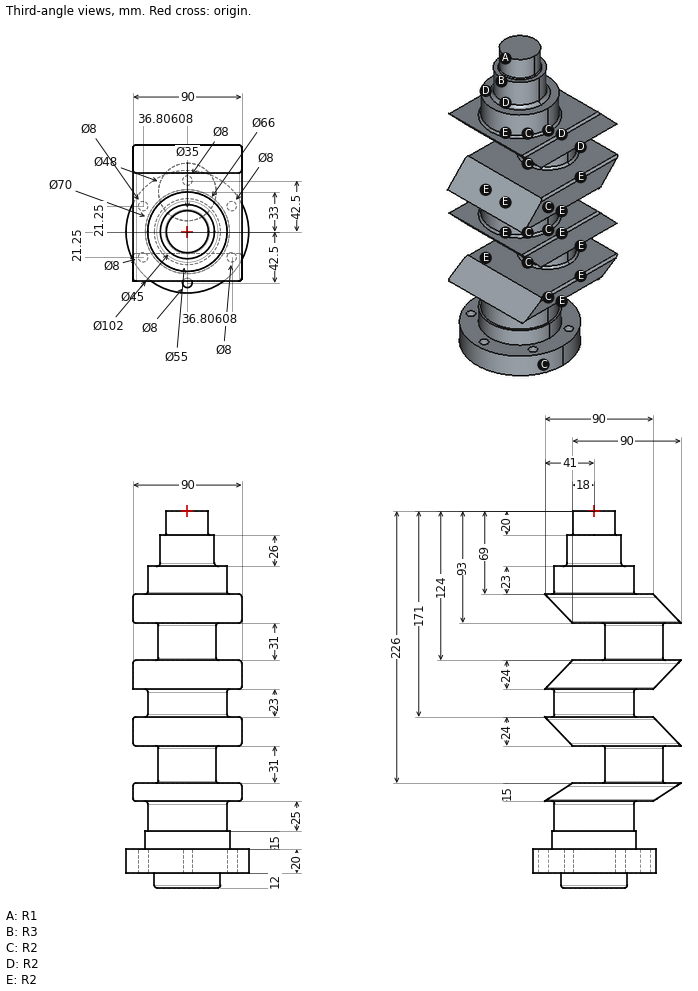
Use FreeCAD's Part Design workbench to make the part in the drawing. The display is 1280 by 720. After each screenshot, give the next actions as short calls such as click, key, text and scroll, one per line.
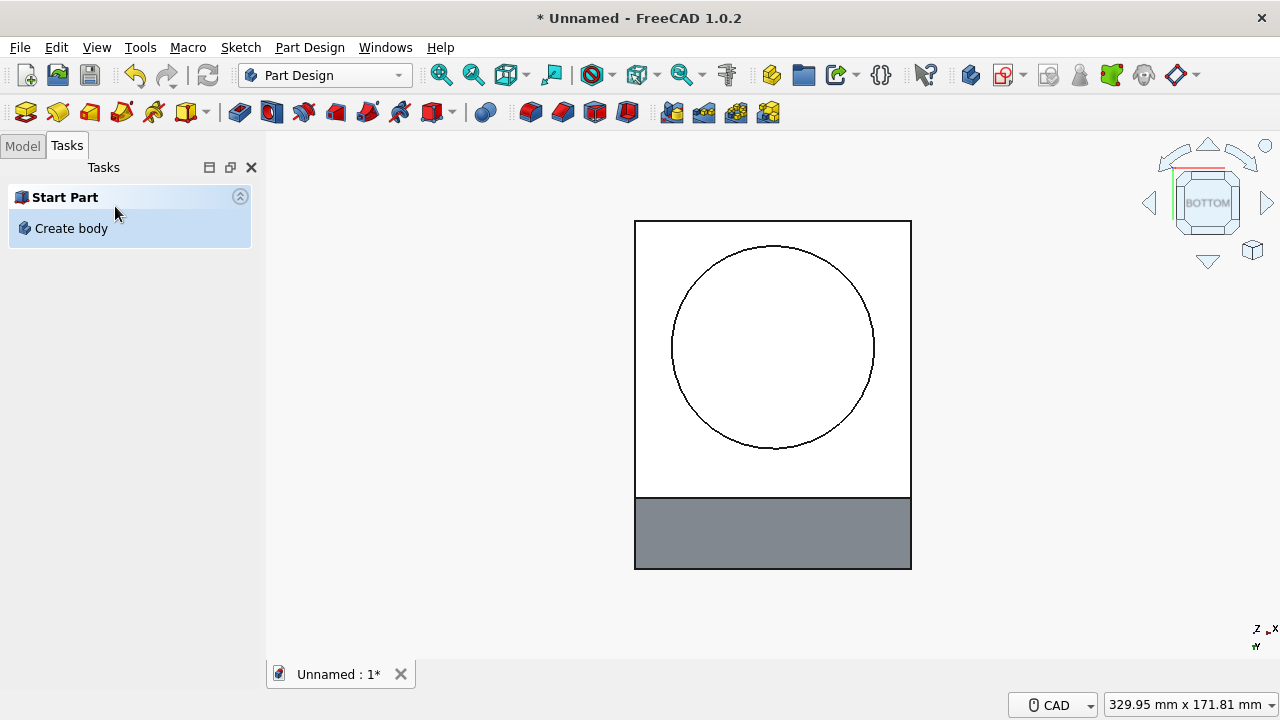
click(1004, 76)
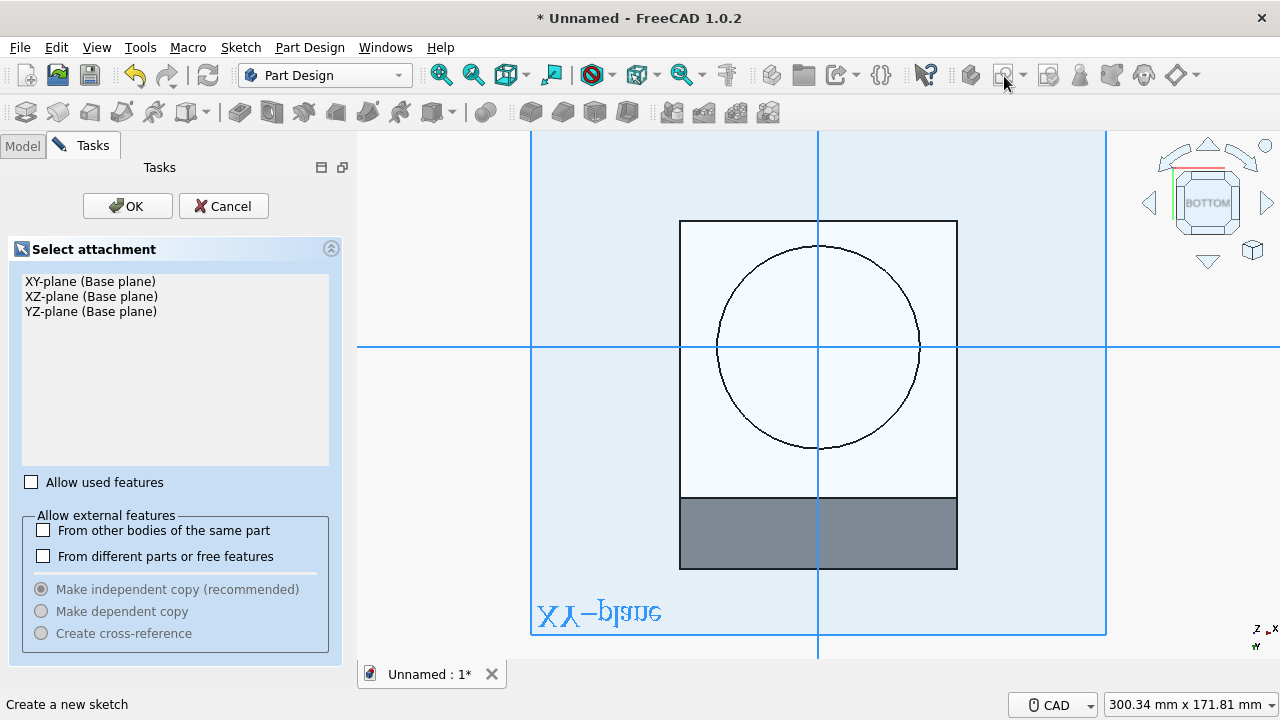
click(82, 312)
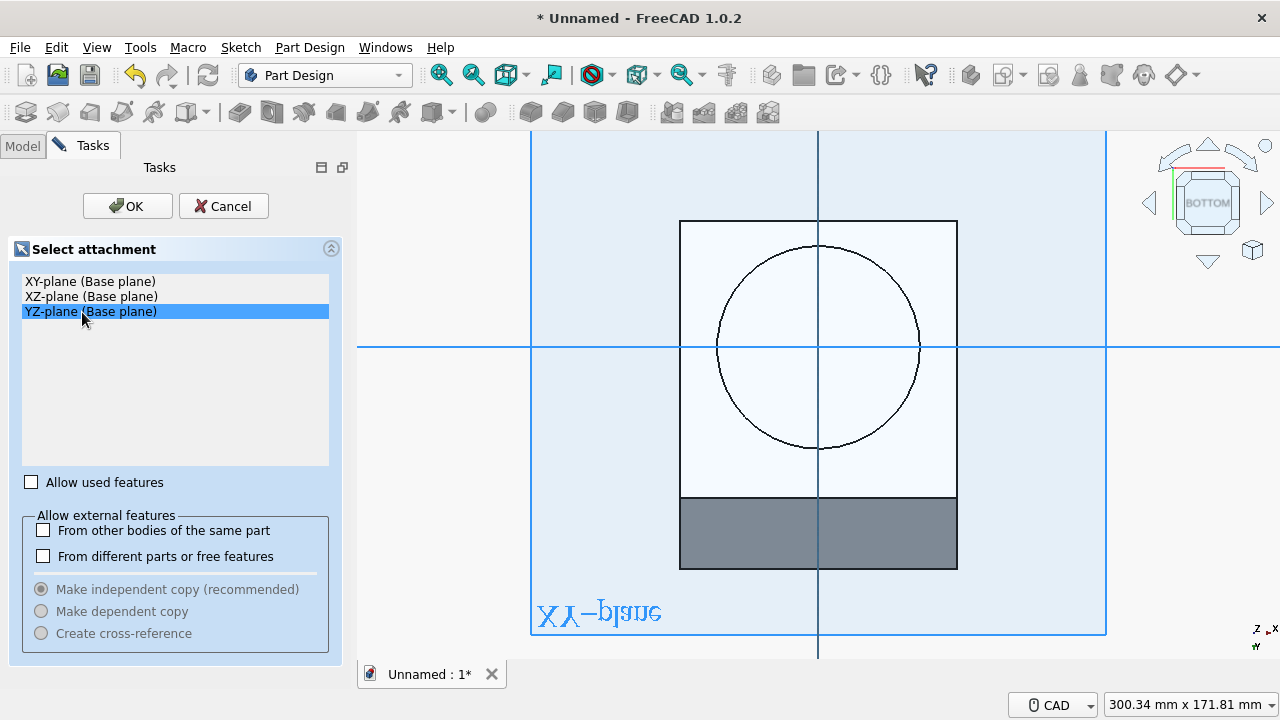
click(128, 206)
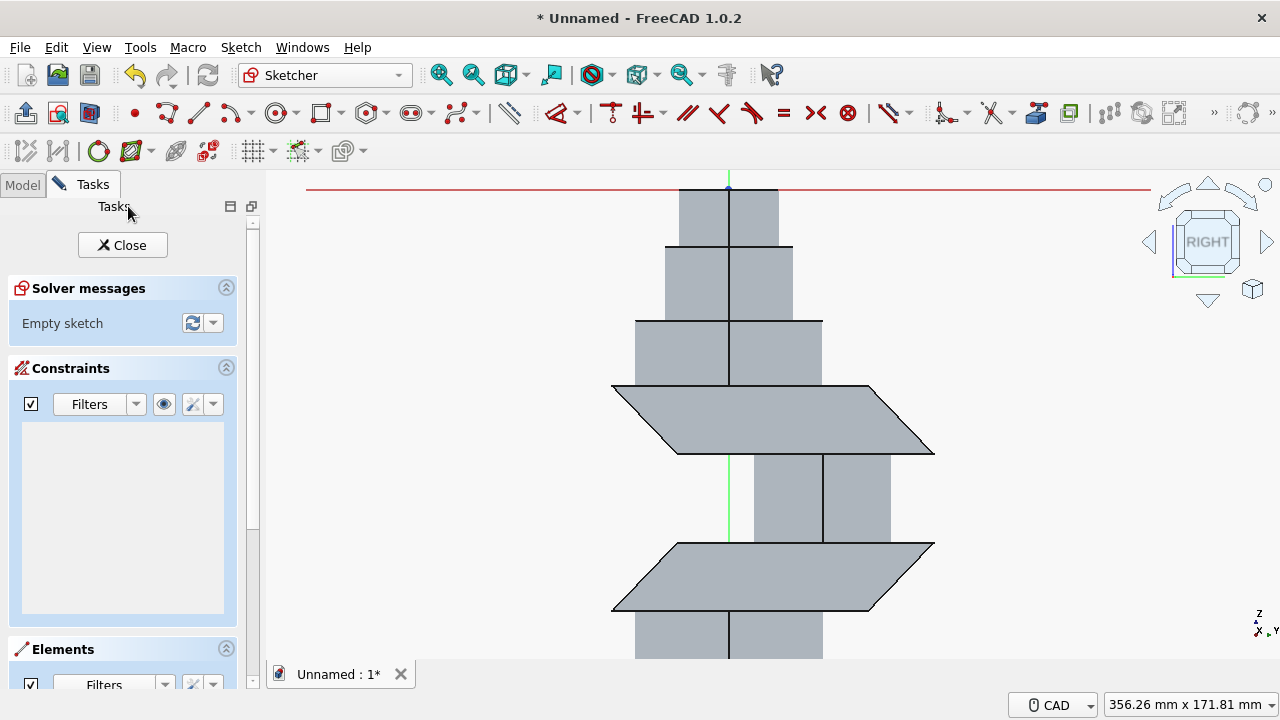
click(90, 114)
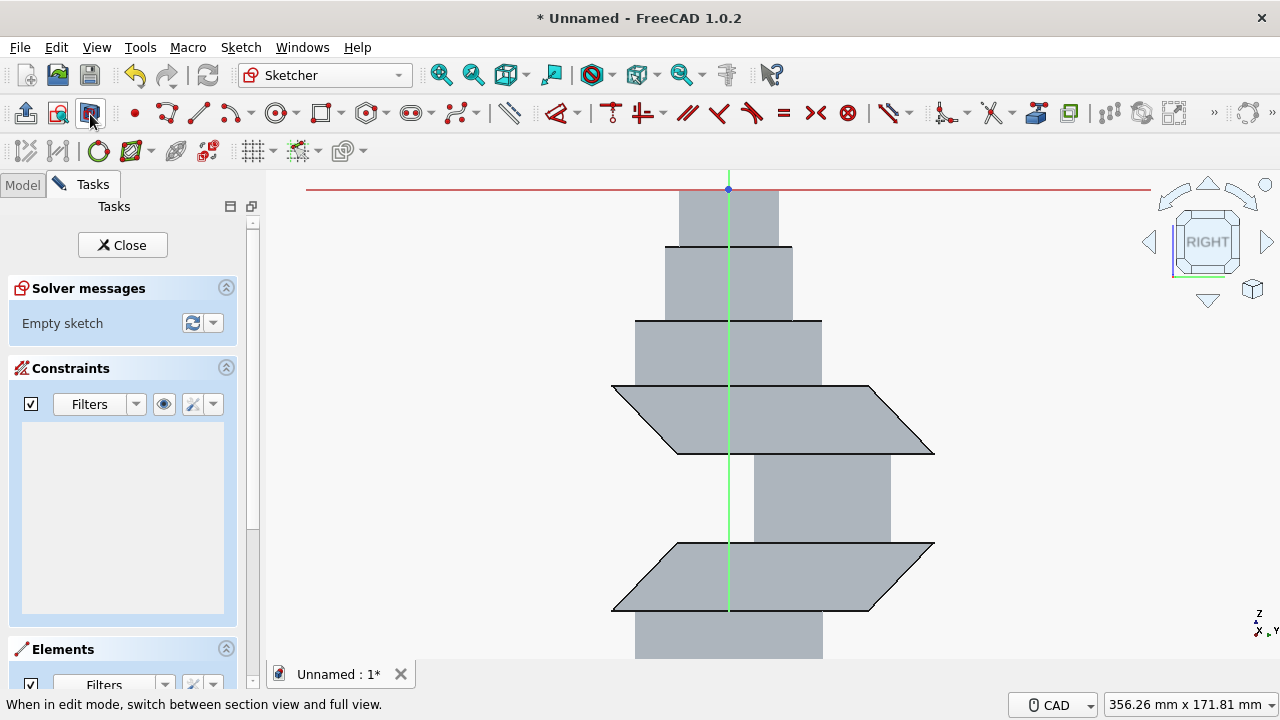
scroll(621, 350, down, 3)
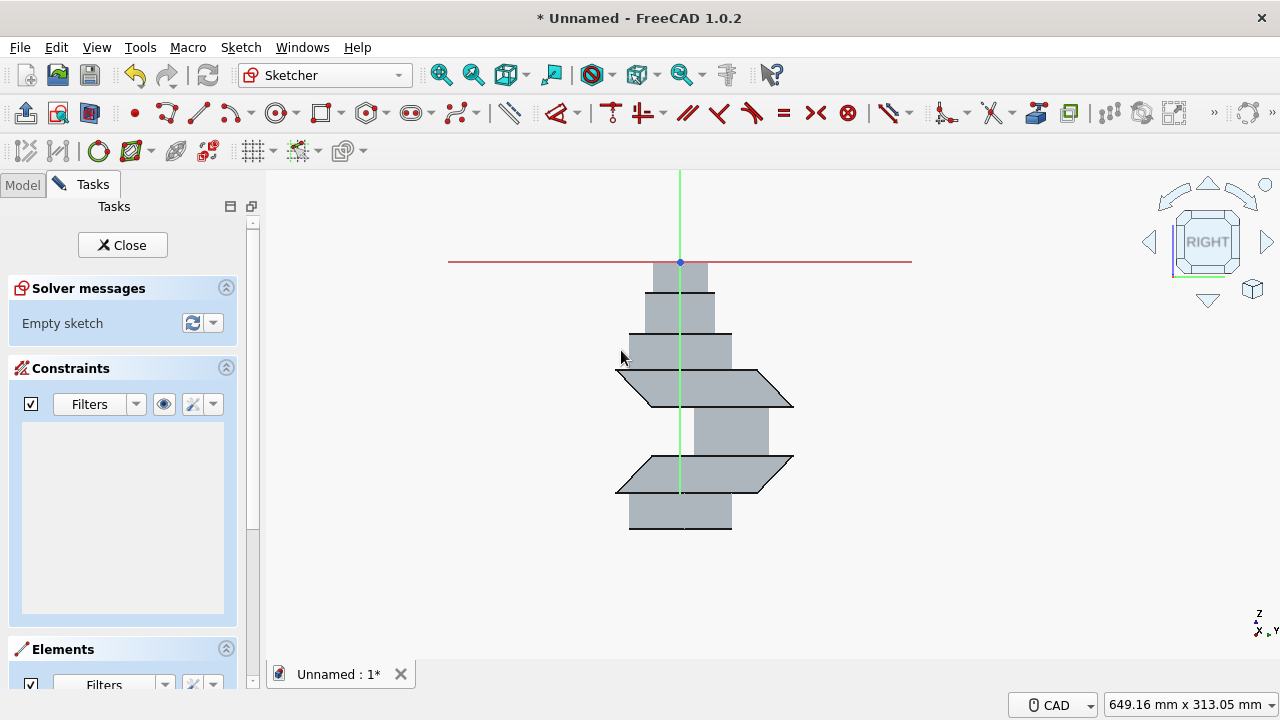
click(168, 114)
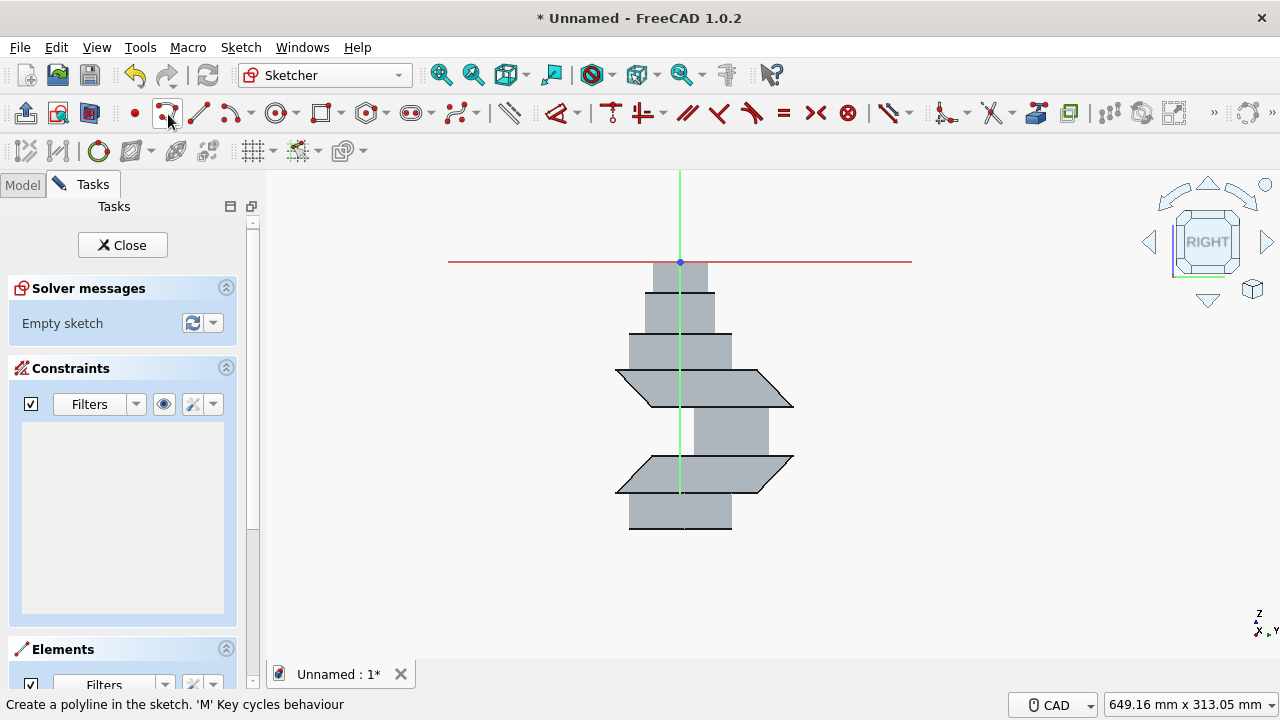
click(616, 529)
click(652, 567)
click(793, 567)
click(757, 529)
click(616, 530)
key(Escape)
key(Escape)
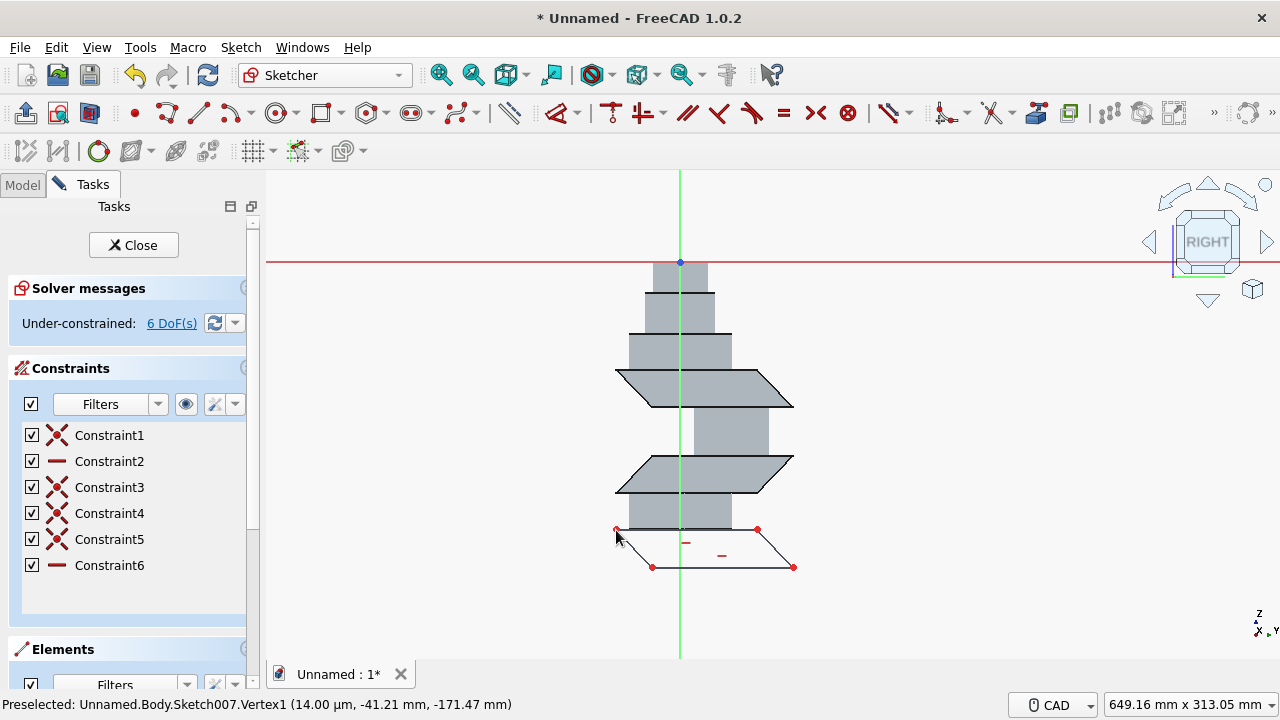
click(556, 114)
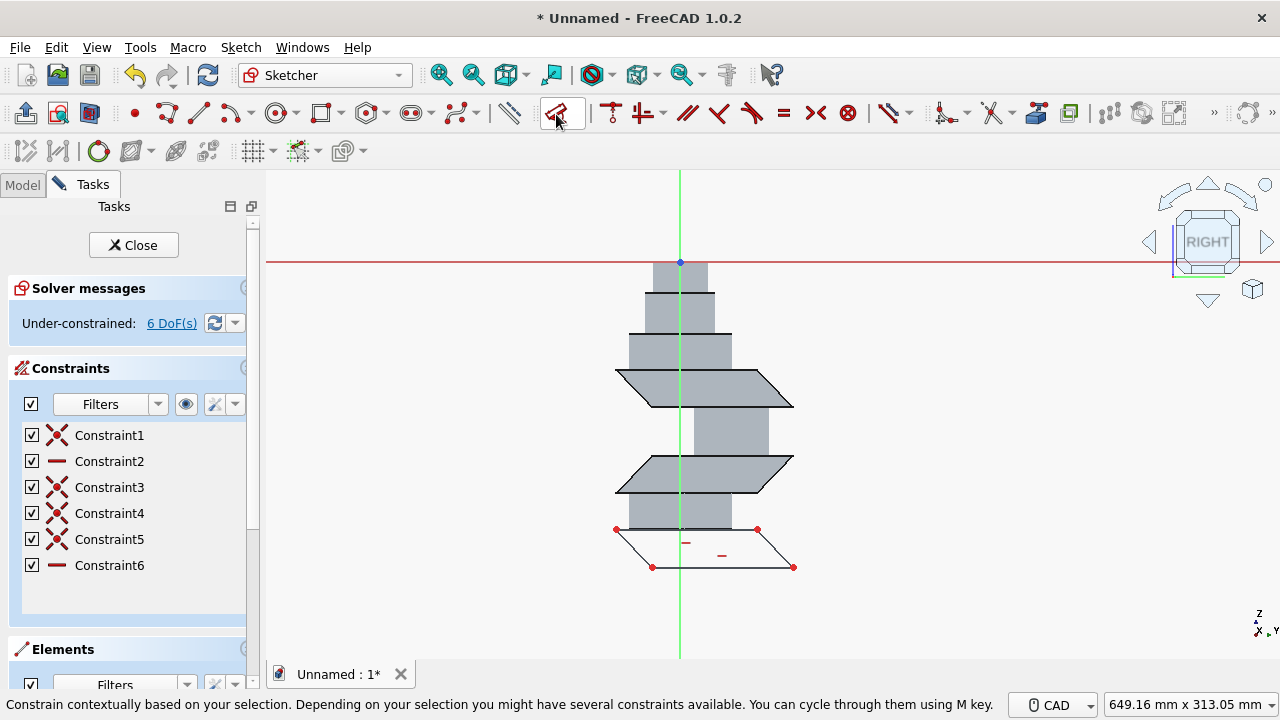
click(694, 568)
click(723, 602)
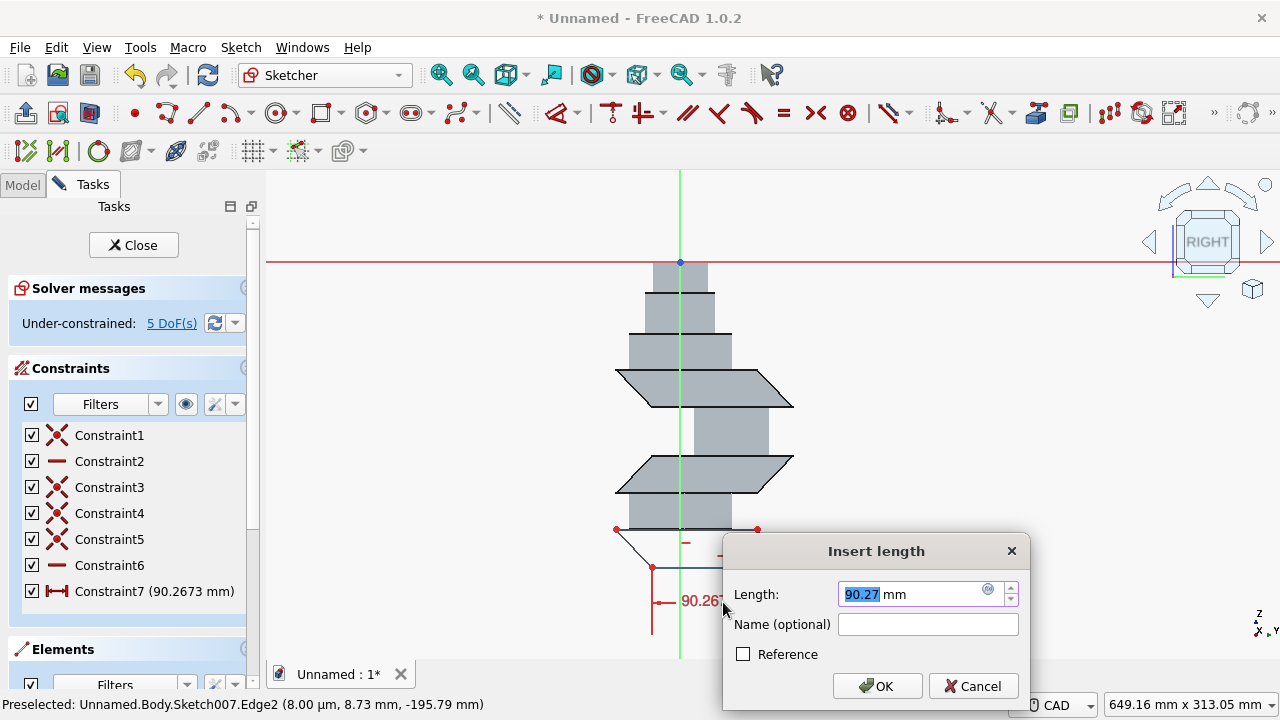
text(90)
key(Return)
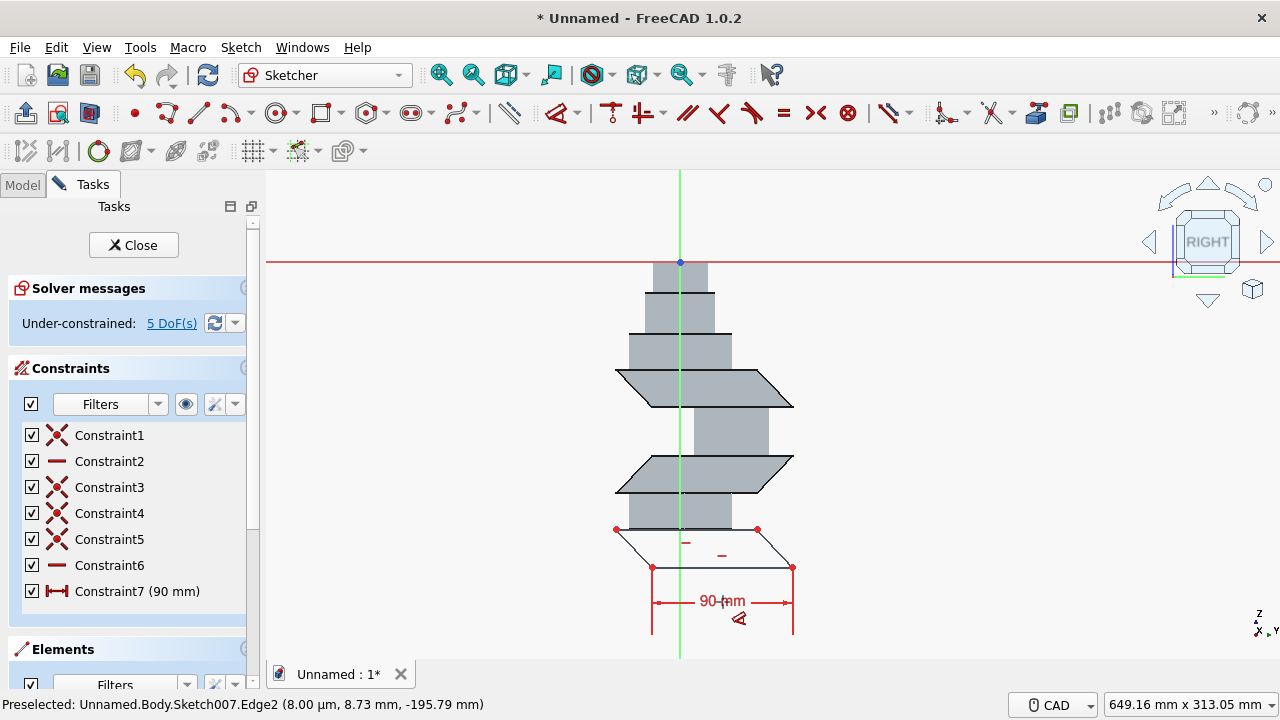
click(715, 530)
click(654, 496)